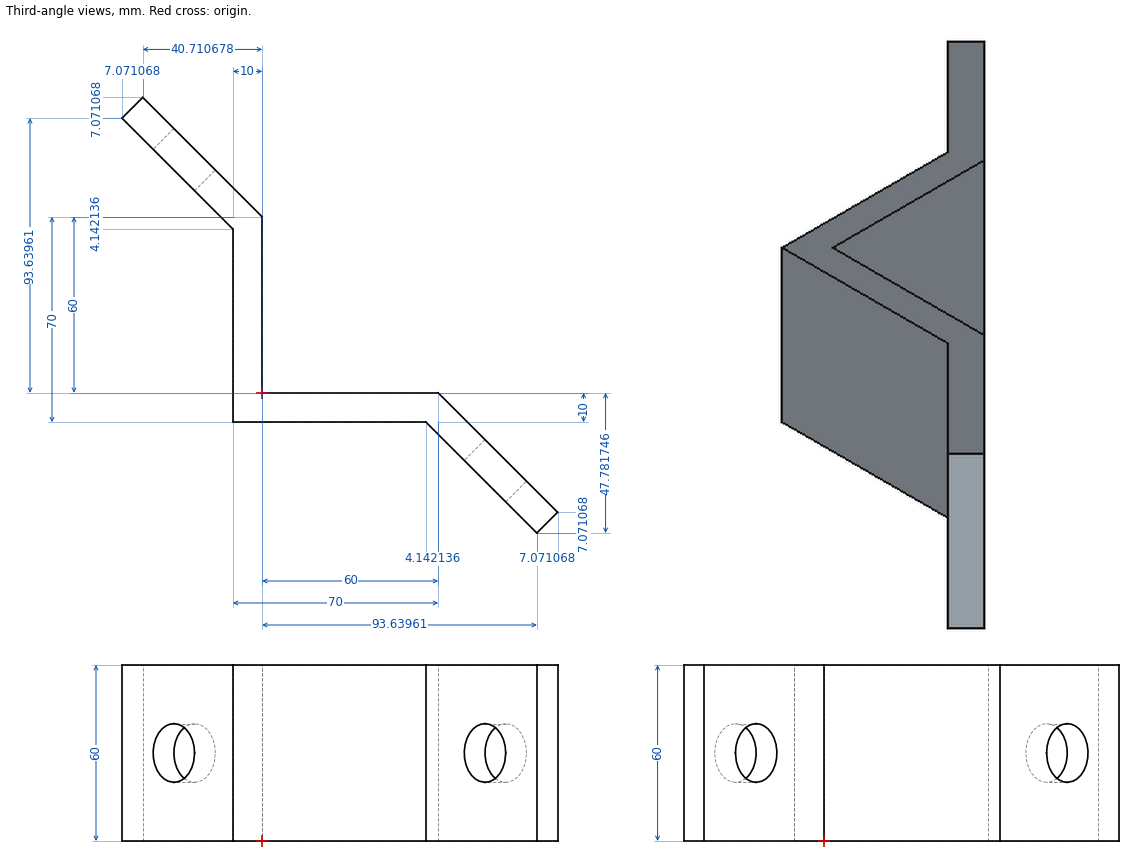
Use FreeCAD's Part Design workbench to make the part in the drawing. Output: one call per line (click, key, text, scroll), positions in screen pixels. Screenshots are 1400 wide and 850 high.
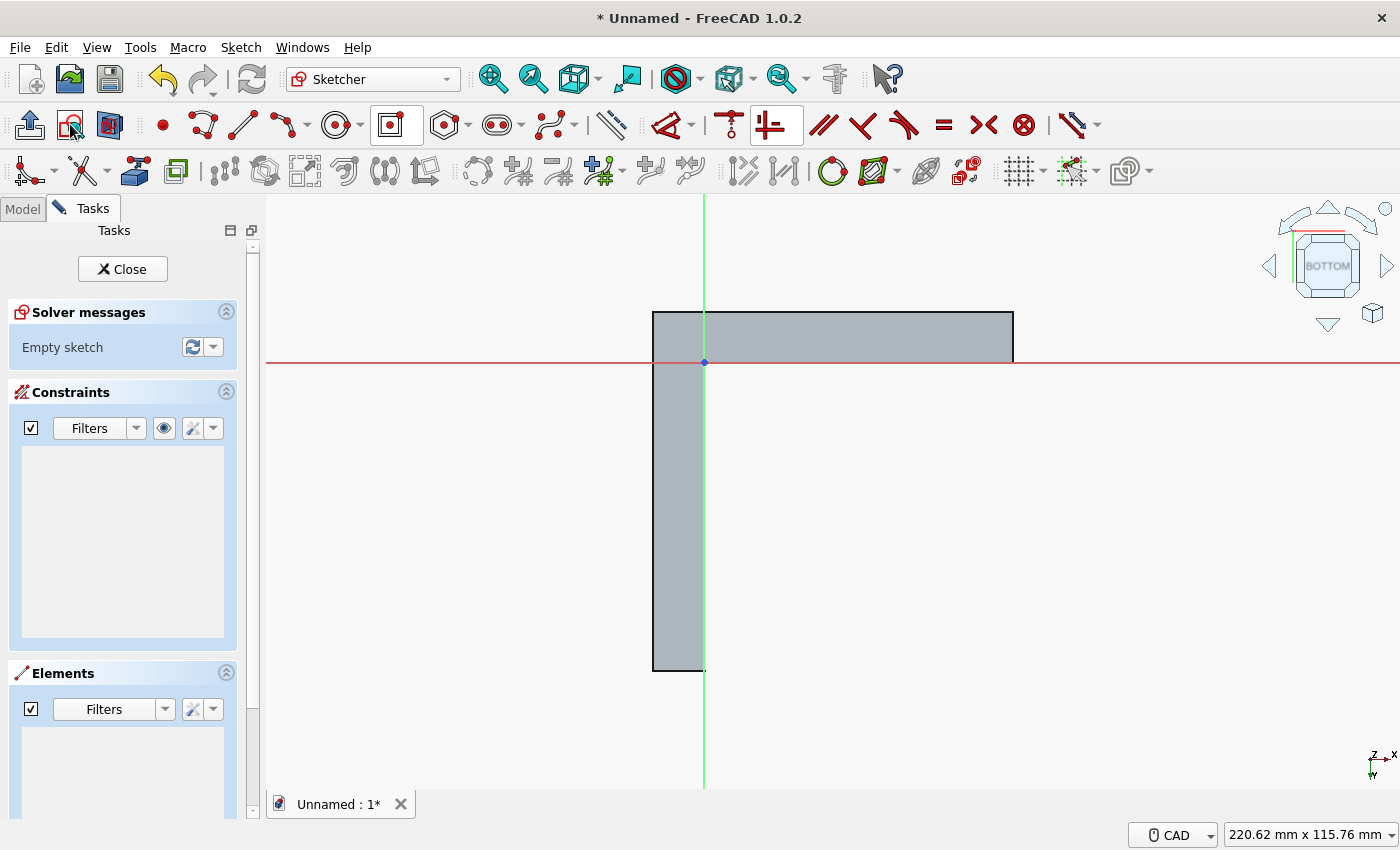
scroll(672, 482, down, 3)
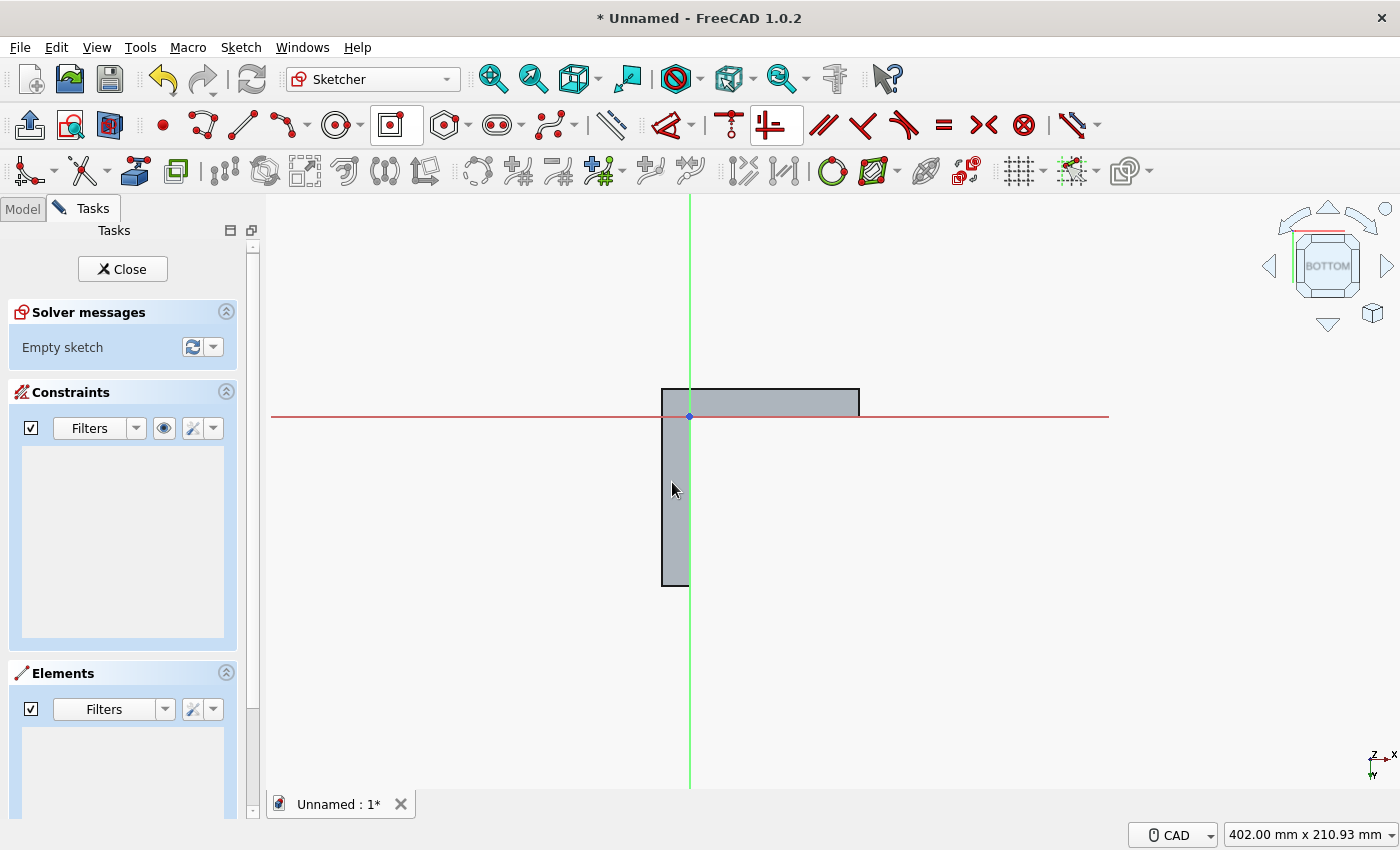
click(204, 126)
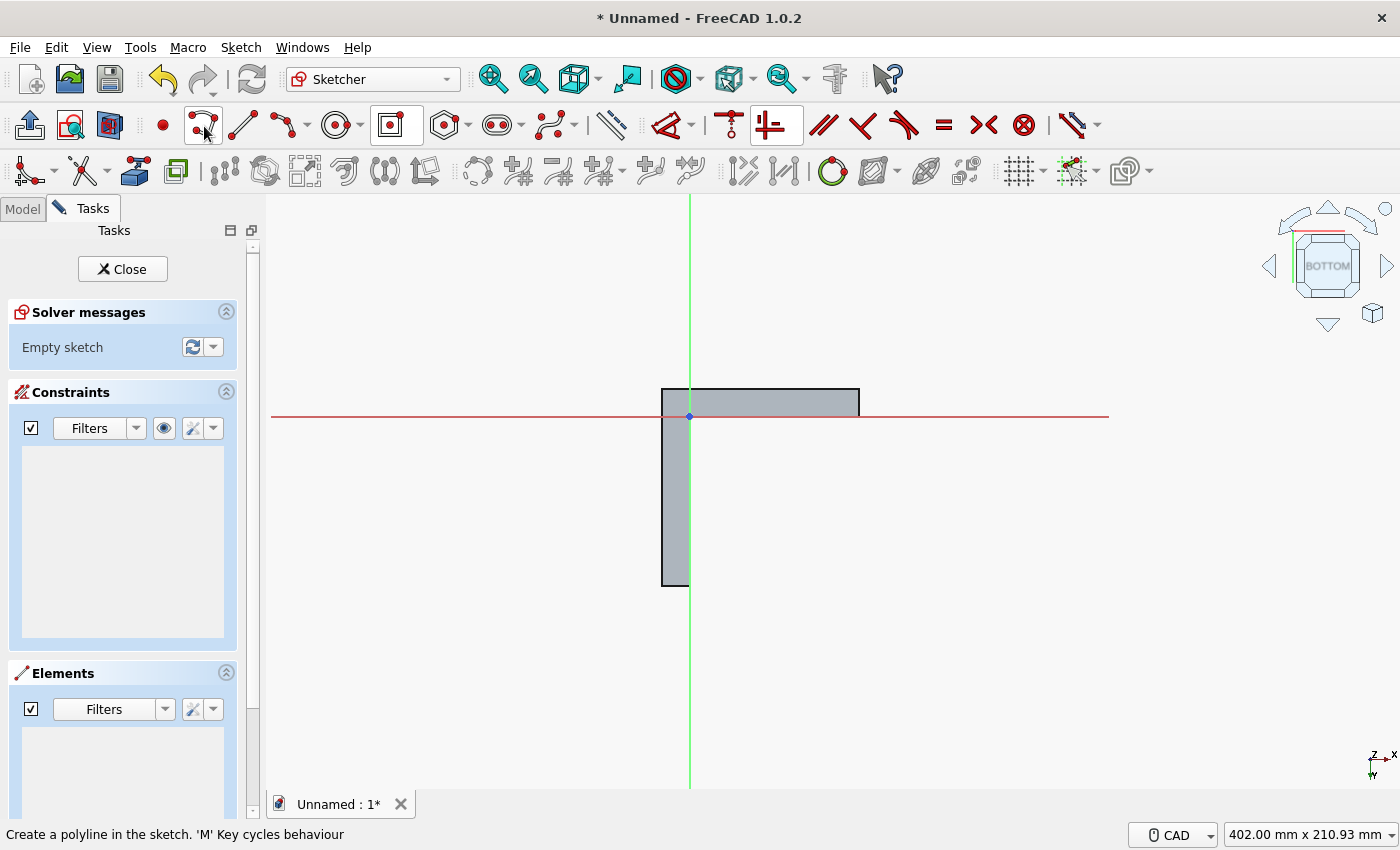
click(662, 574)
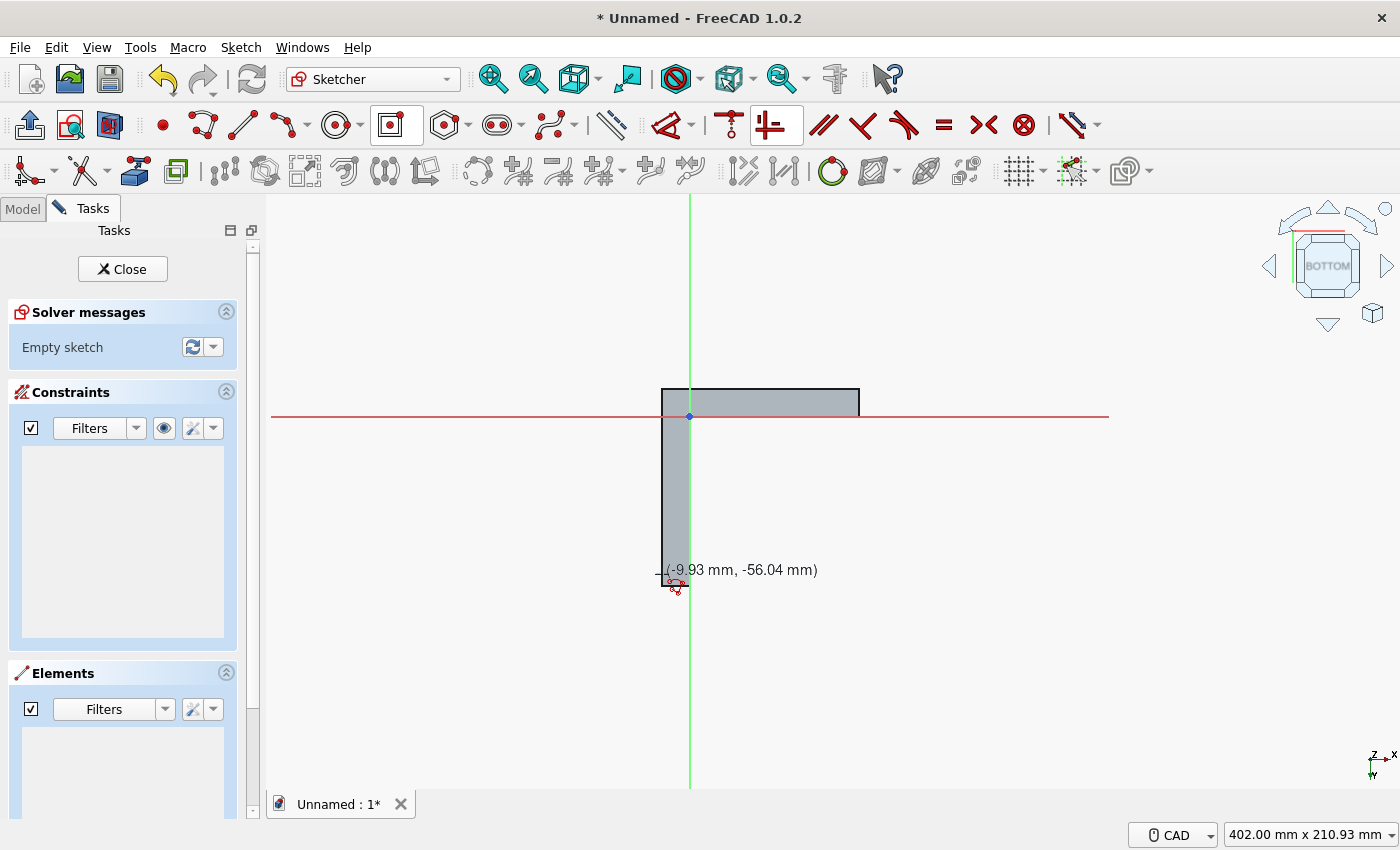
scroll(662, 586, up, 2)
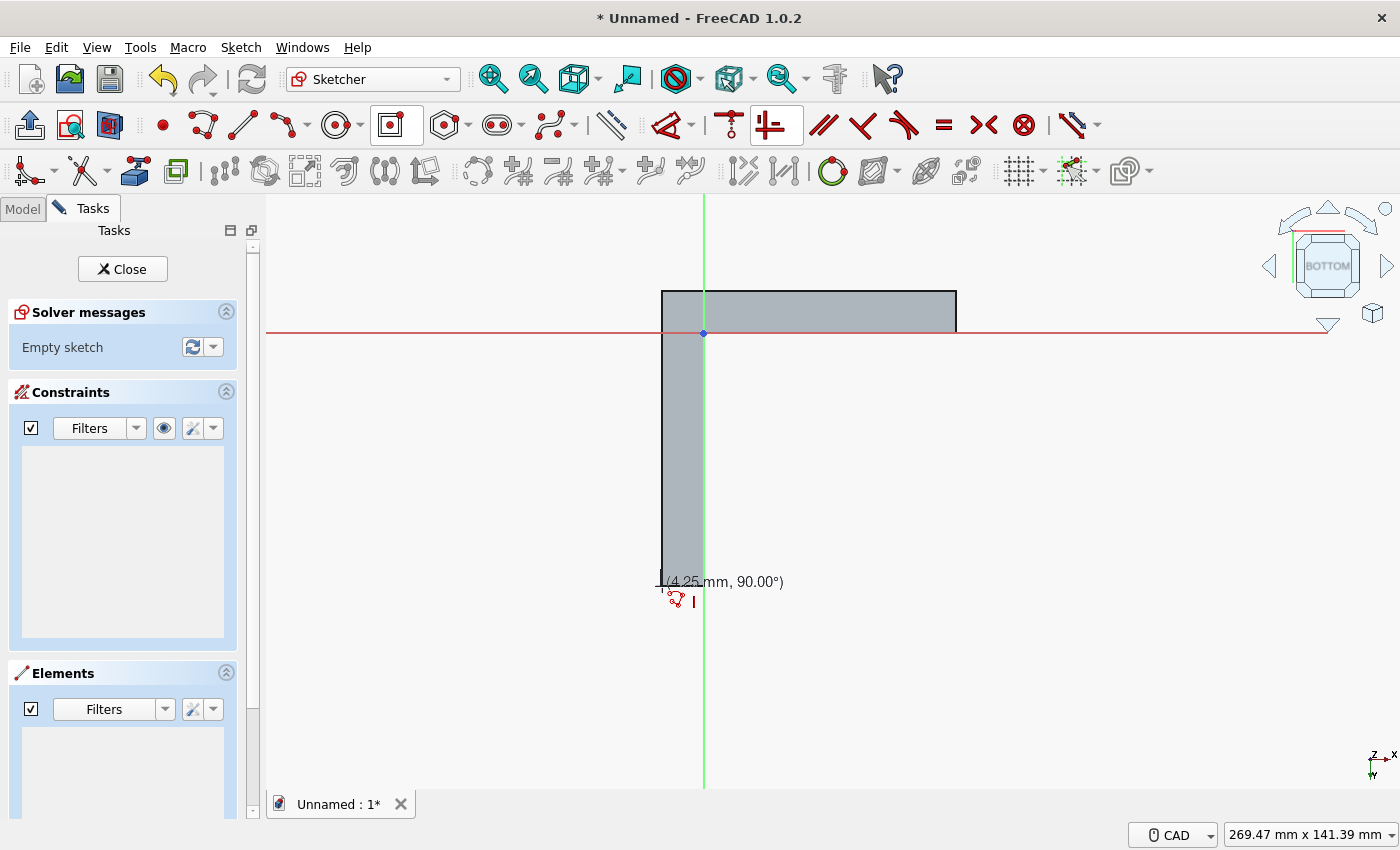
click(662, 586)
click(704, 586)
click(532, 757)
click(503, 727)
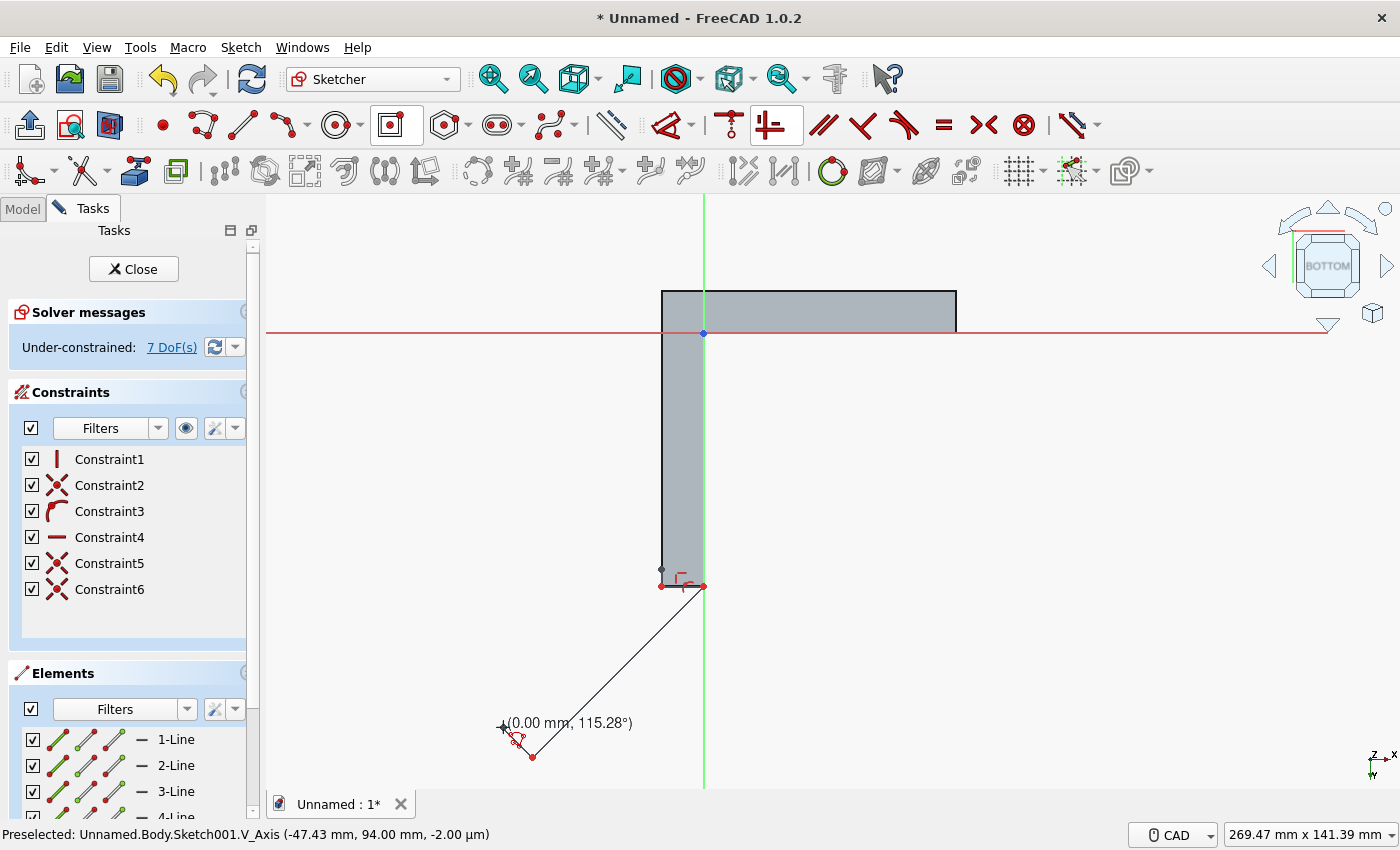
scroll(662, 568, up, 3)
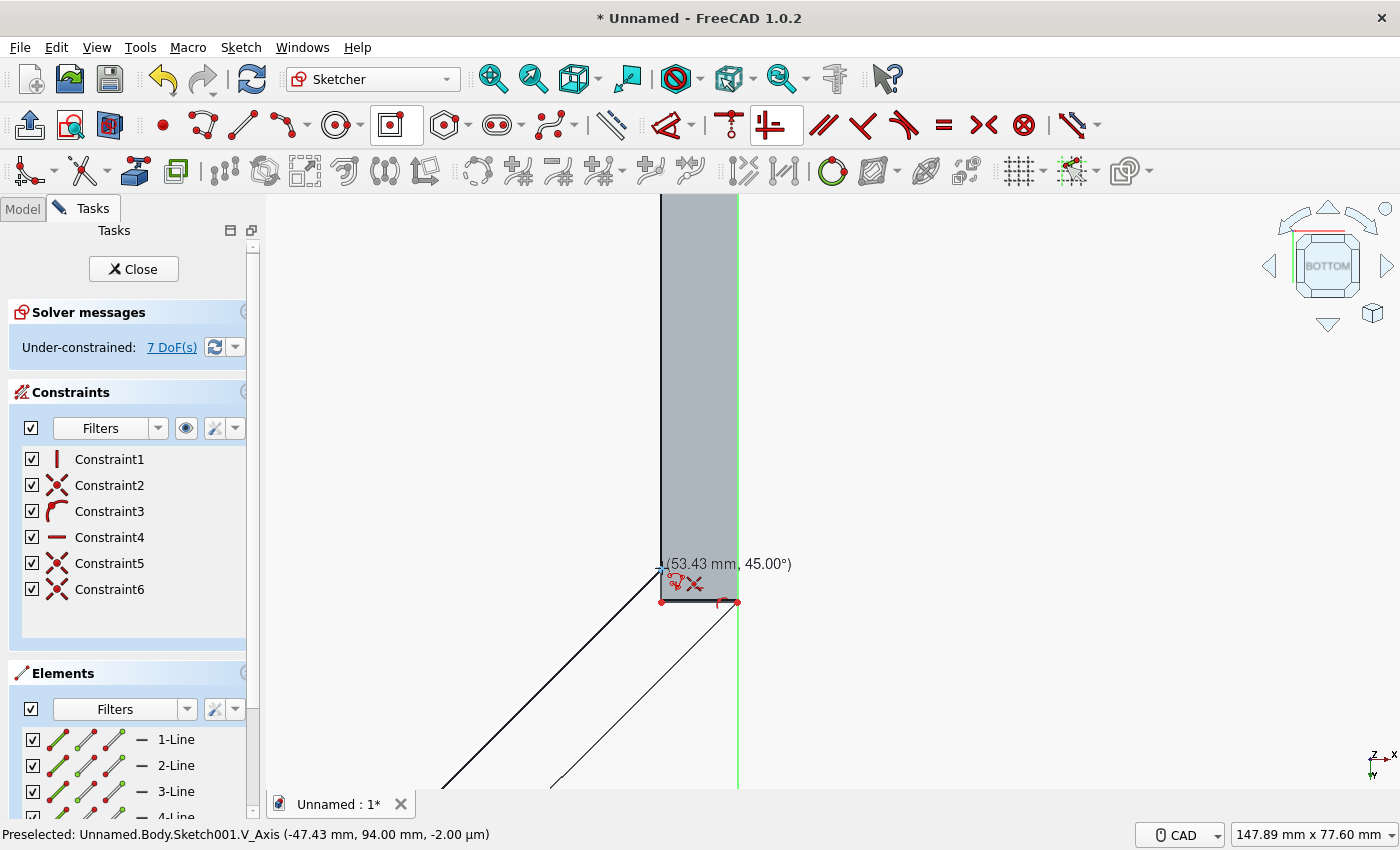
click(661, 570)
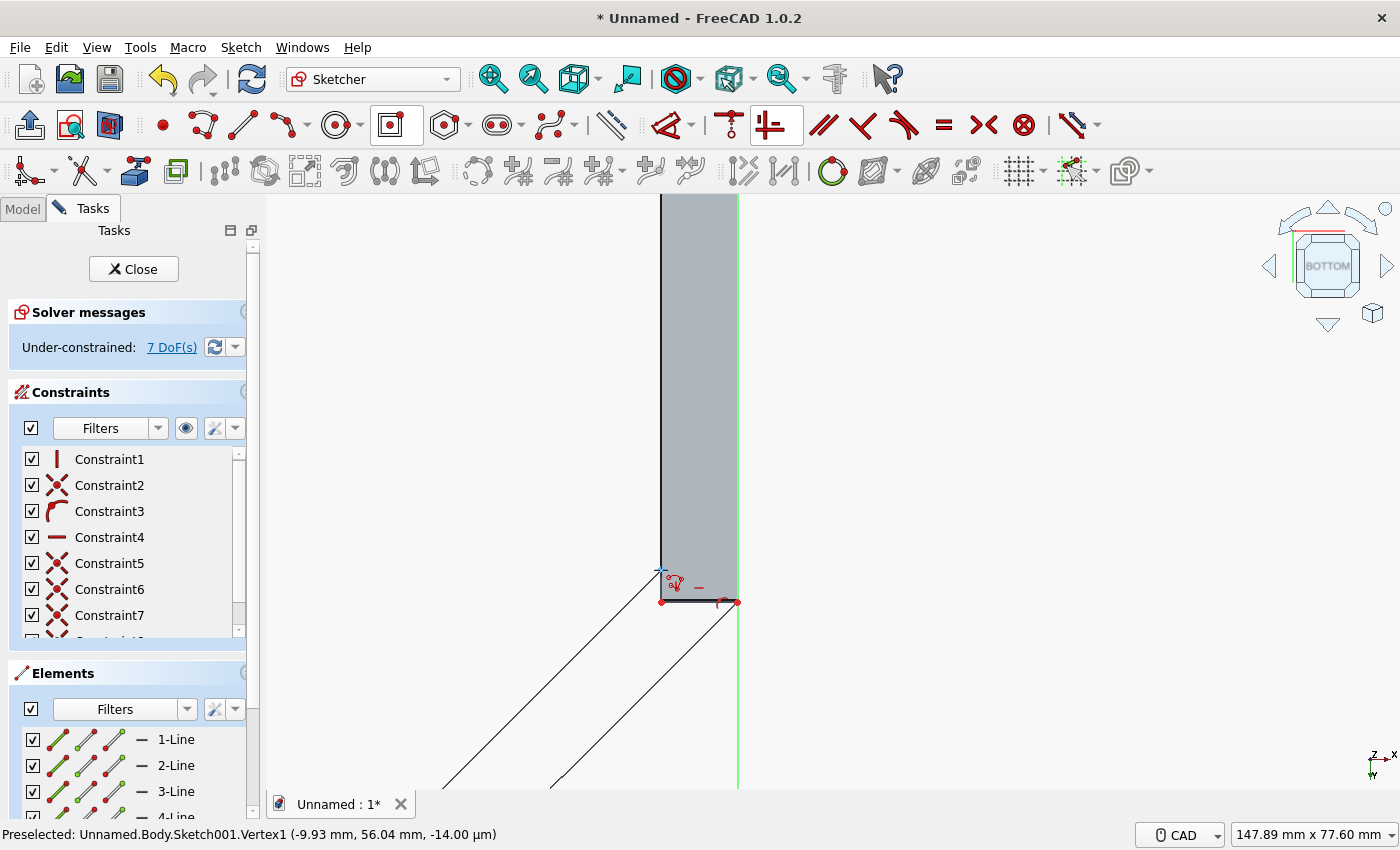
scroll(662, 578, down, 5)